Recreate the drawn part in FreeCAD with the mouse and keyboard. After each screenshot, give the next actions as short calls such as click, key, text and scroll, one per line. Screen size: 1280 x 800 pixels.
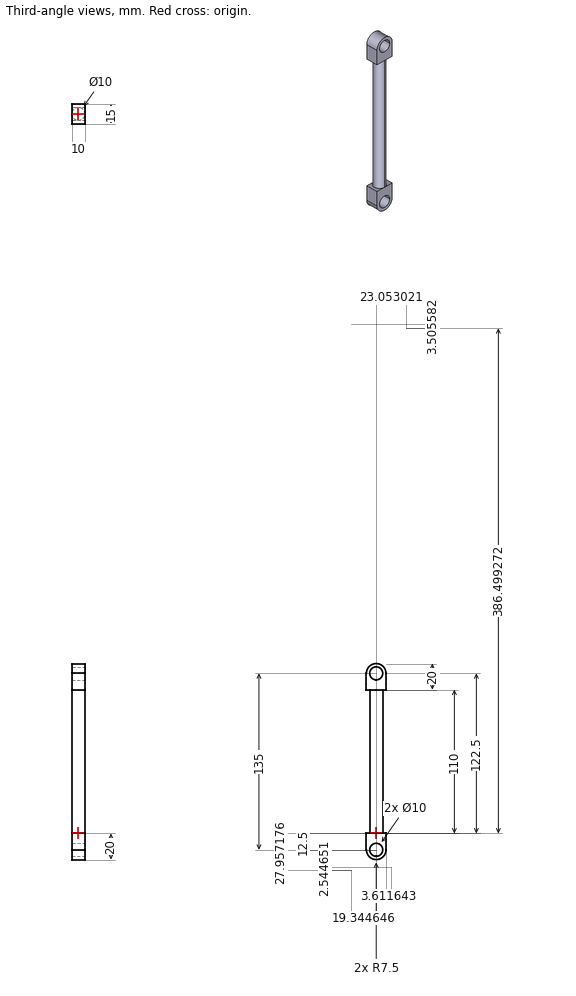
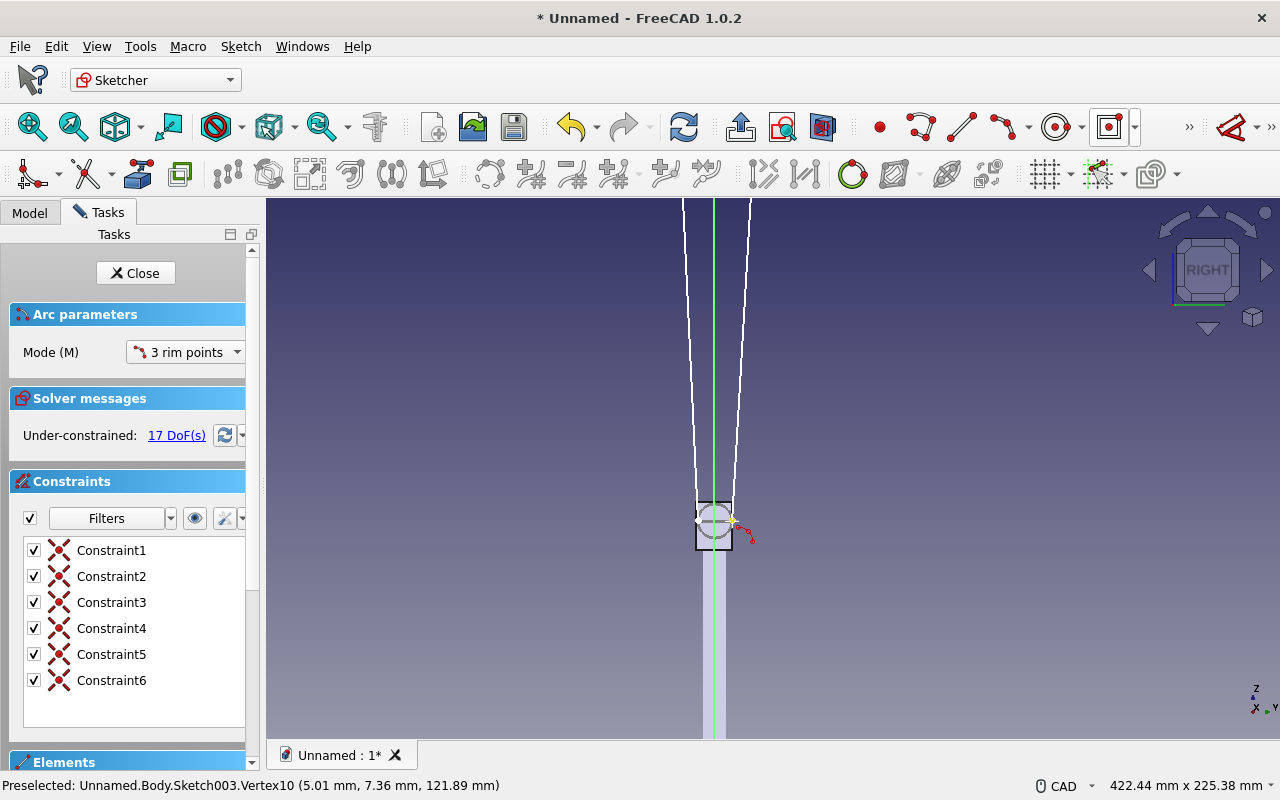
scroll(725, 505, up, 4)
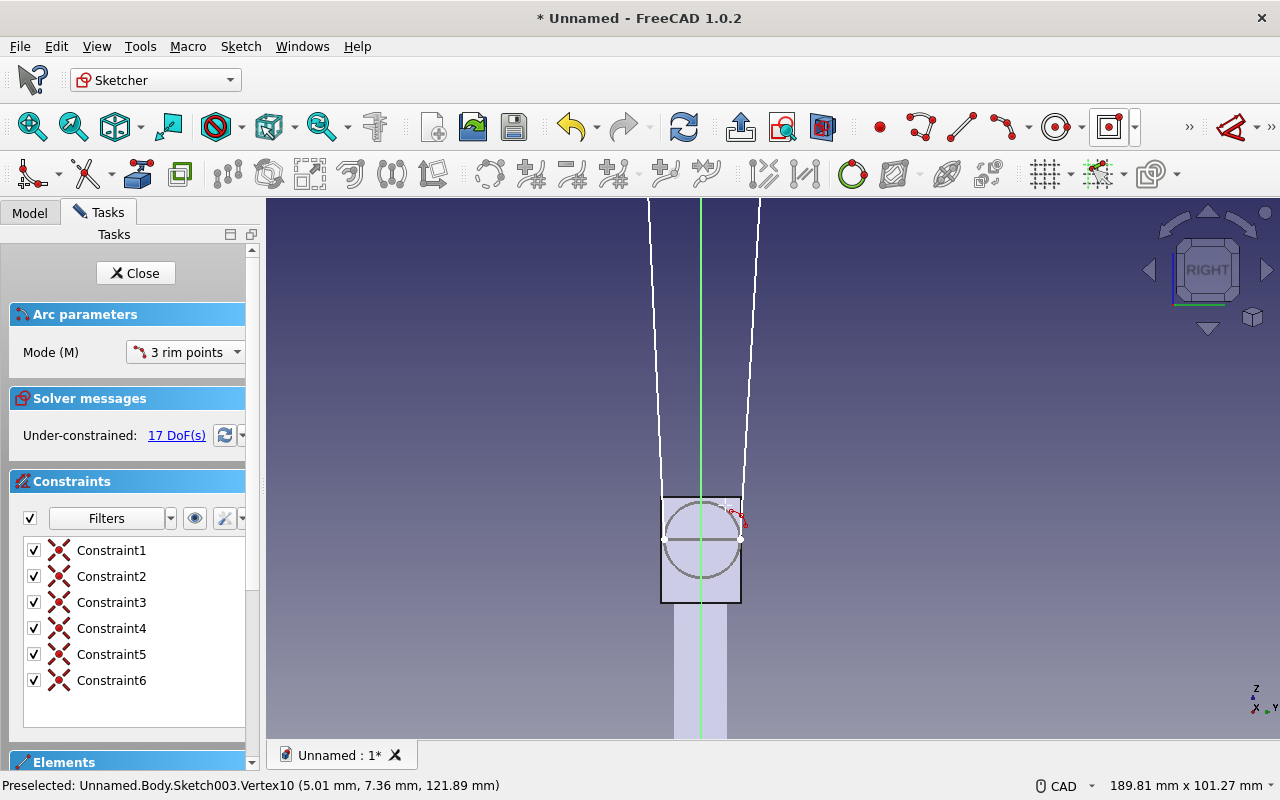
click(724, 504)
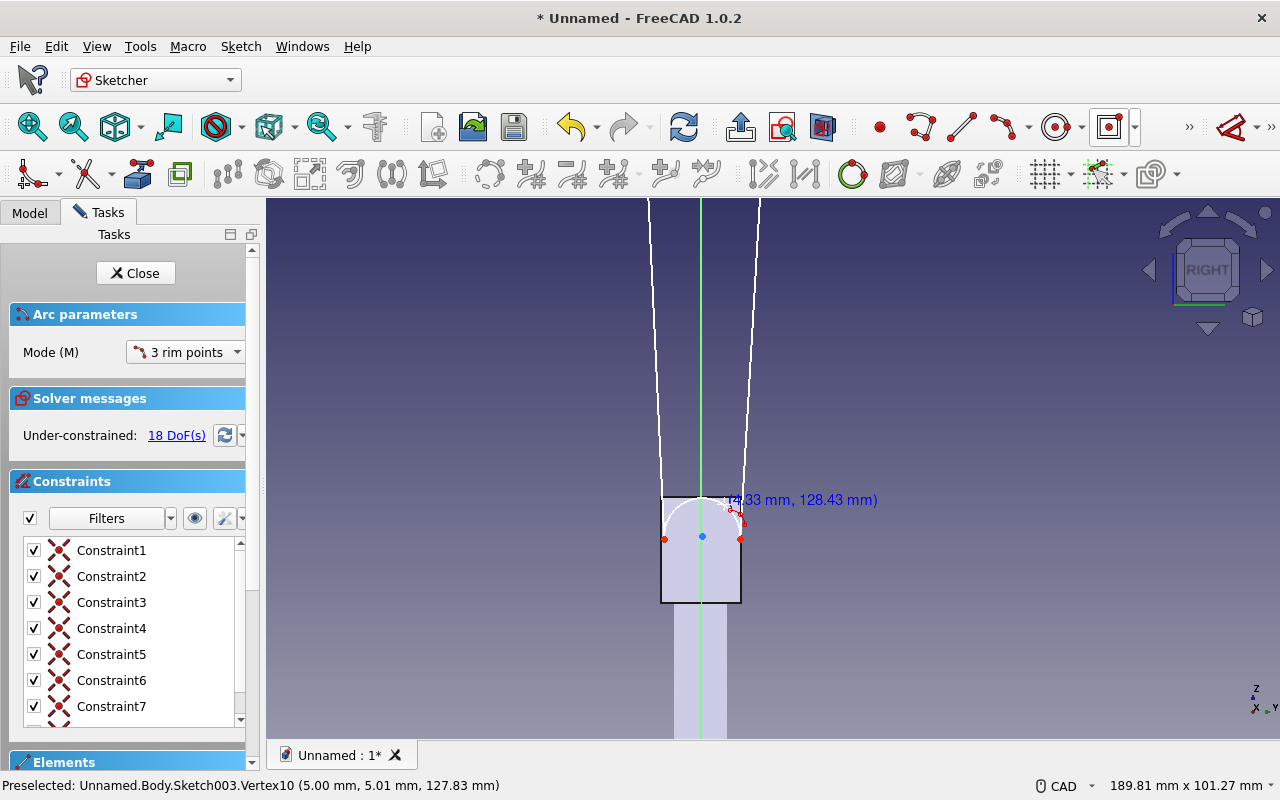
click(1056, 128)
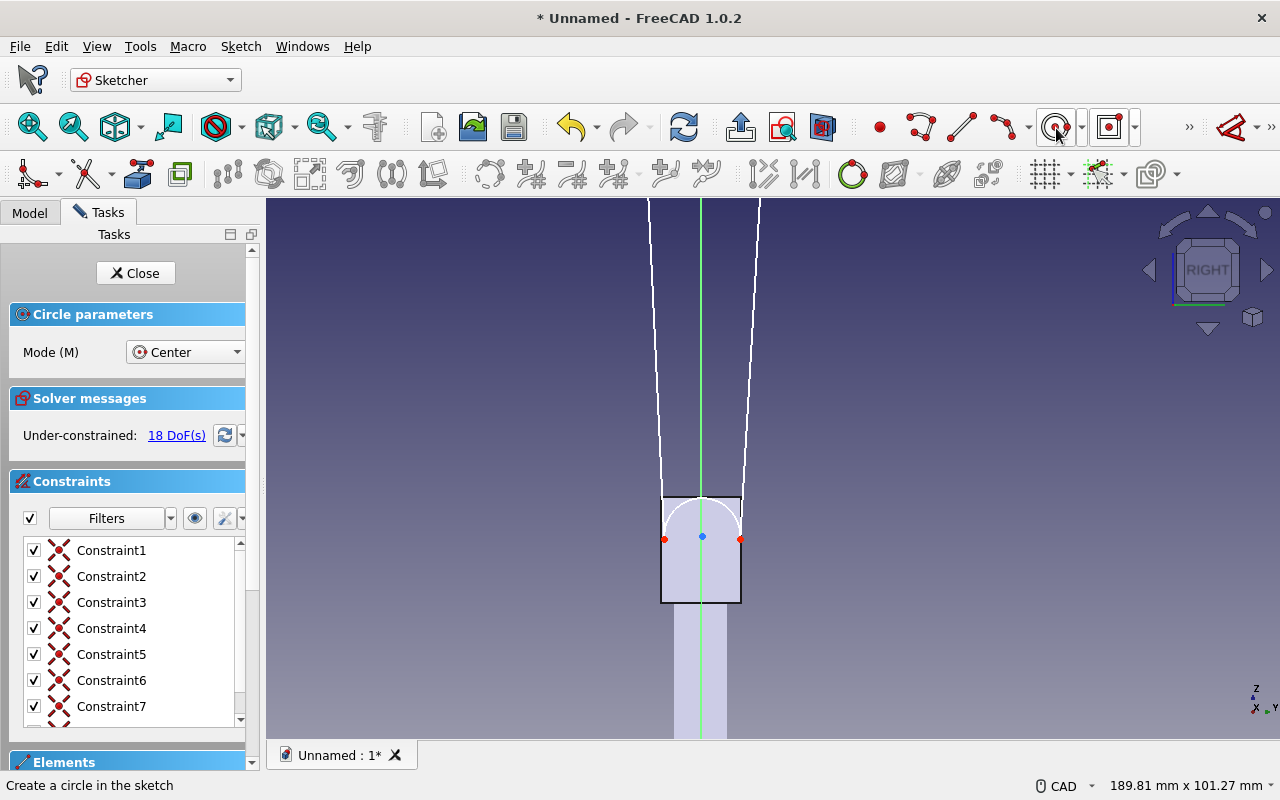
scroll(703, 517, down, 9)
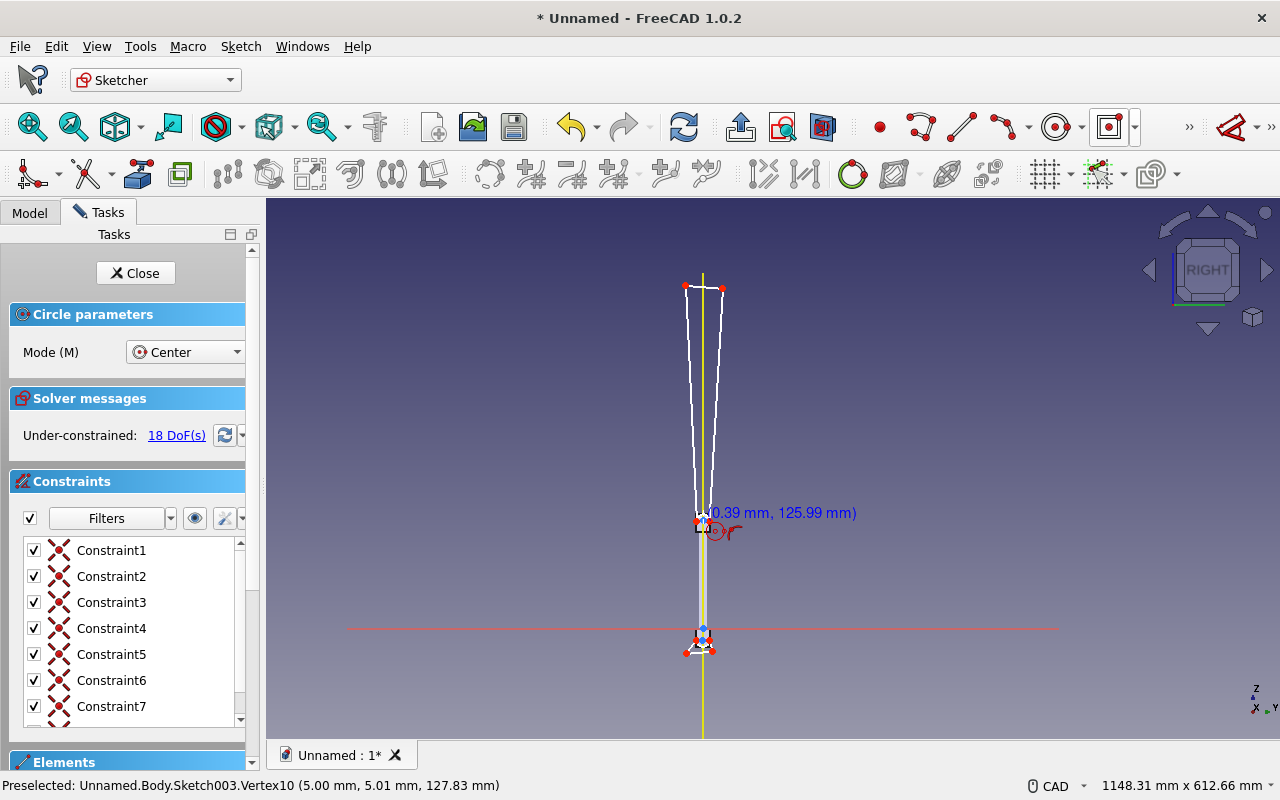
scroll(703, 640, up, 9)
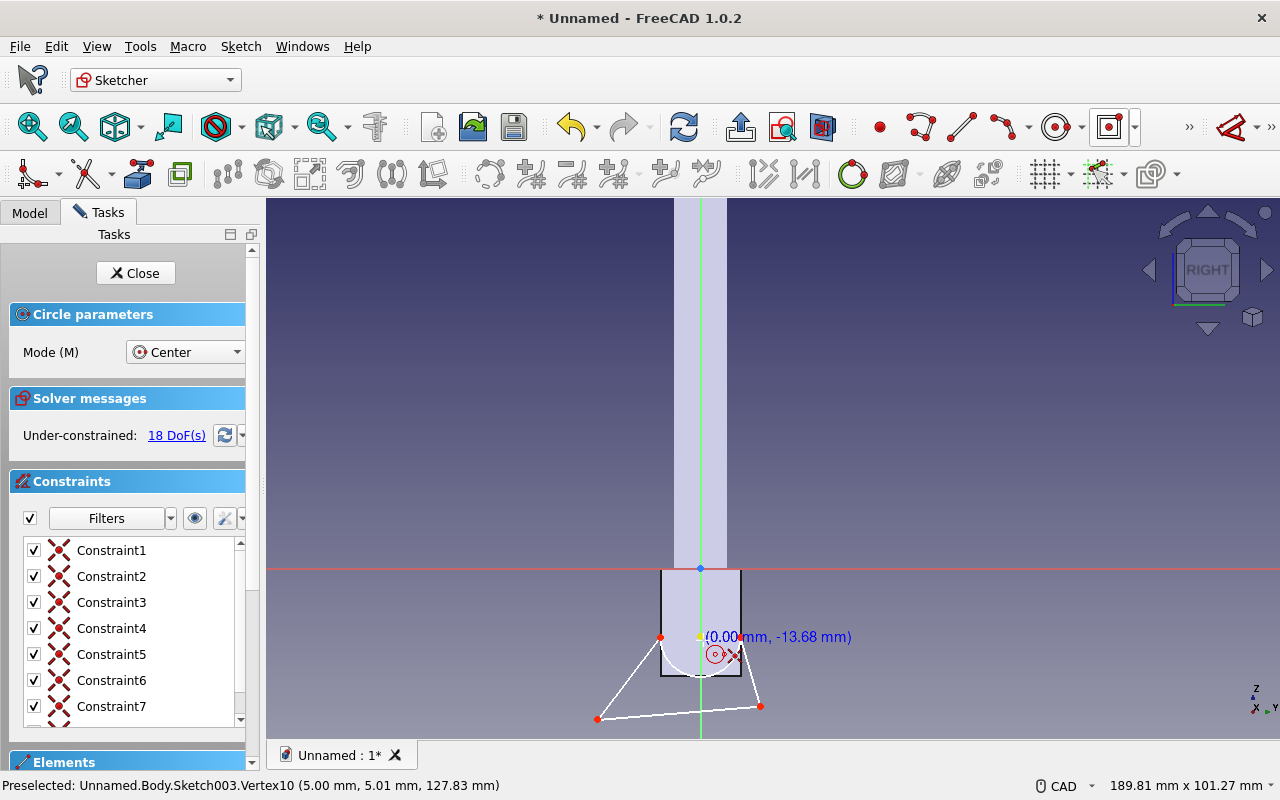
click(701, 636)
move(720, 617)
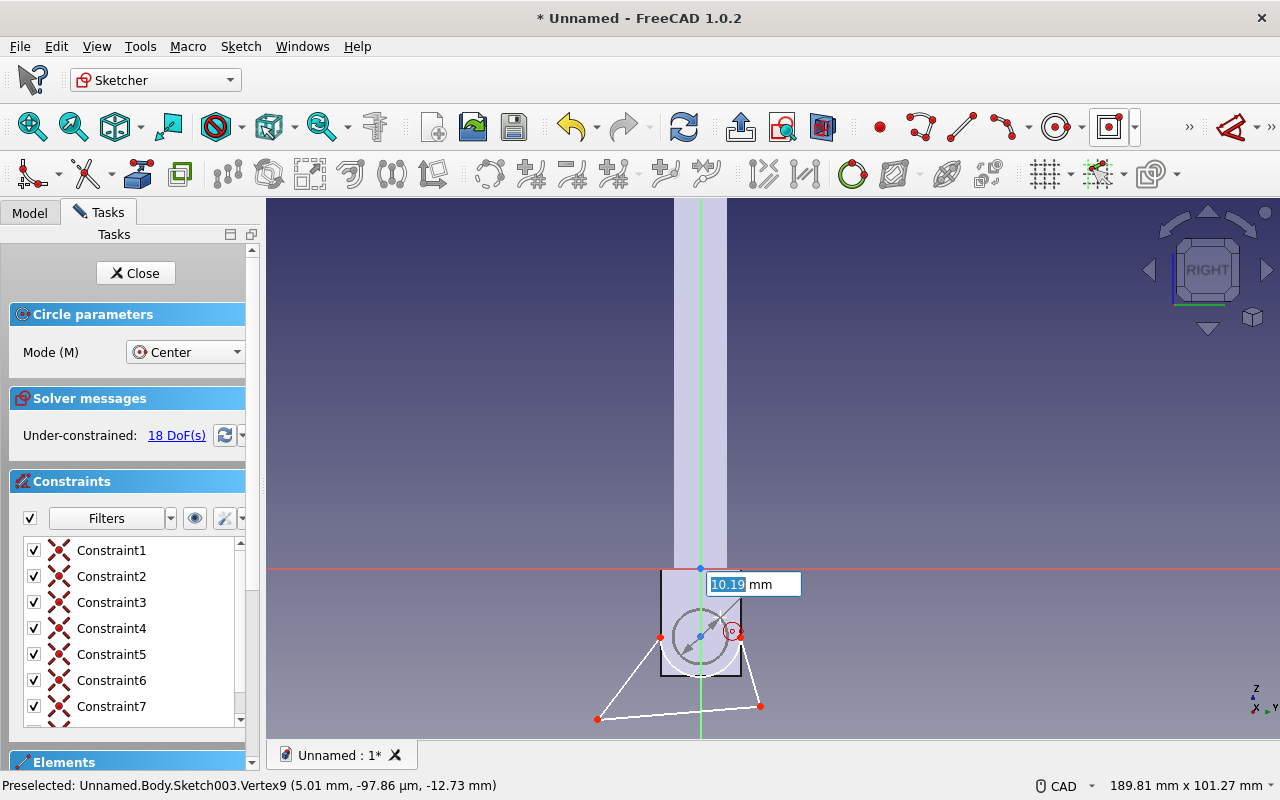
text(10)
key(Return)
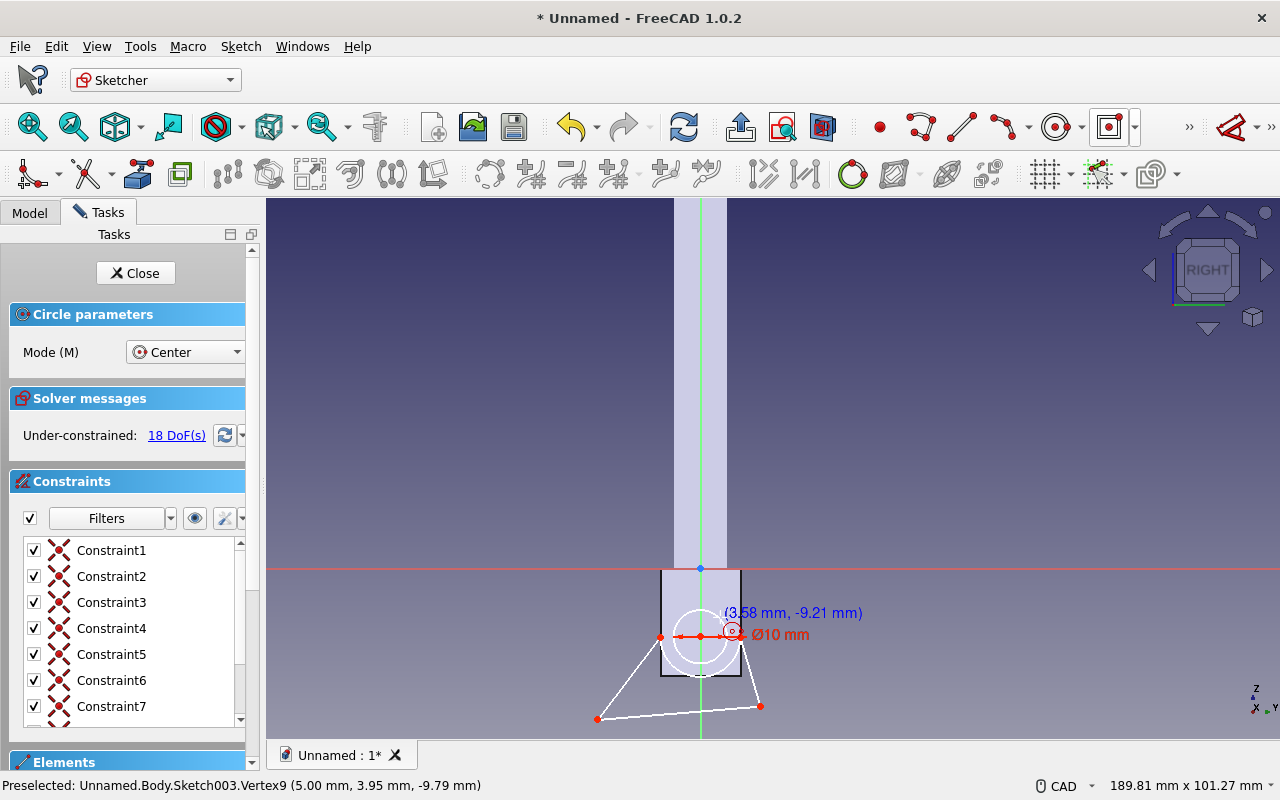
scroll(703, 640, down, 9)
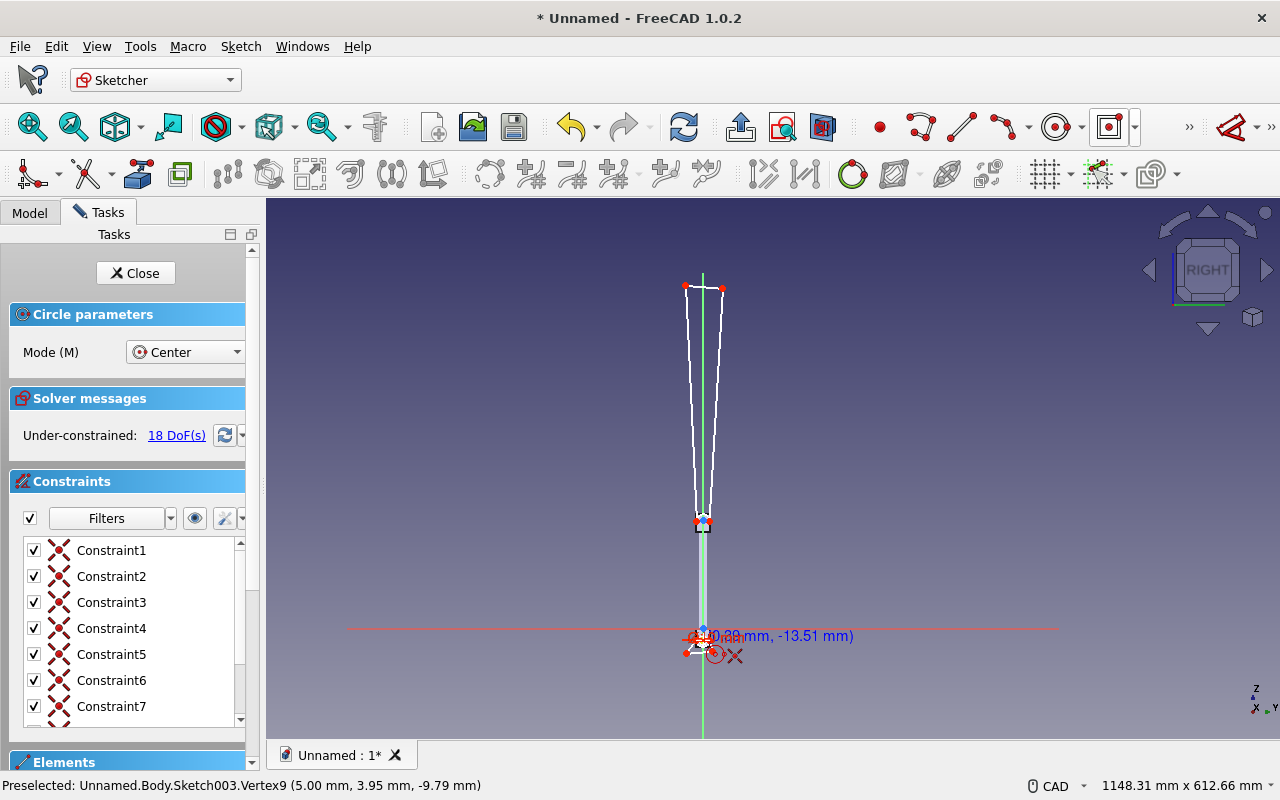
scroll(703, 521, up, 9)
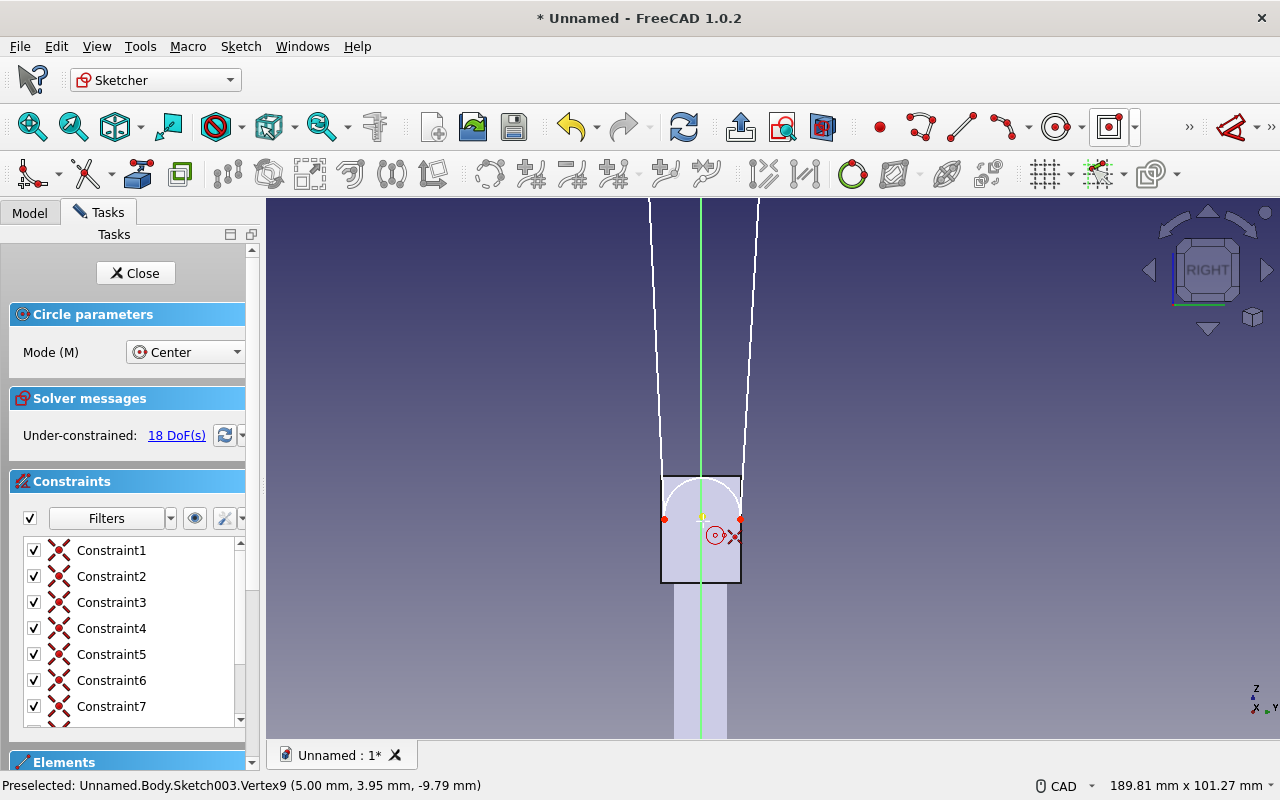
click(701, 516)
move(720, 535)